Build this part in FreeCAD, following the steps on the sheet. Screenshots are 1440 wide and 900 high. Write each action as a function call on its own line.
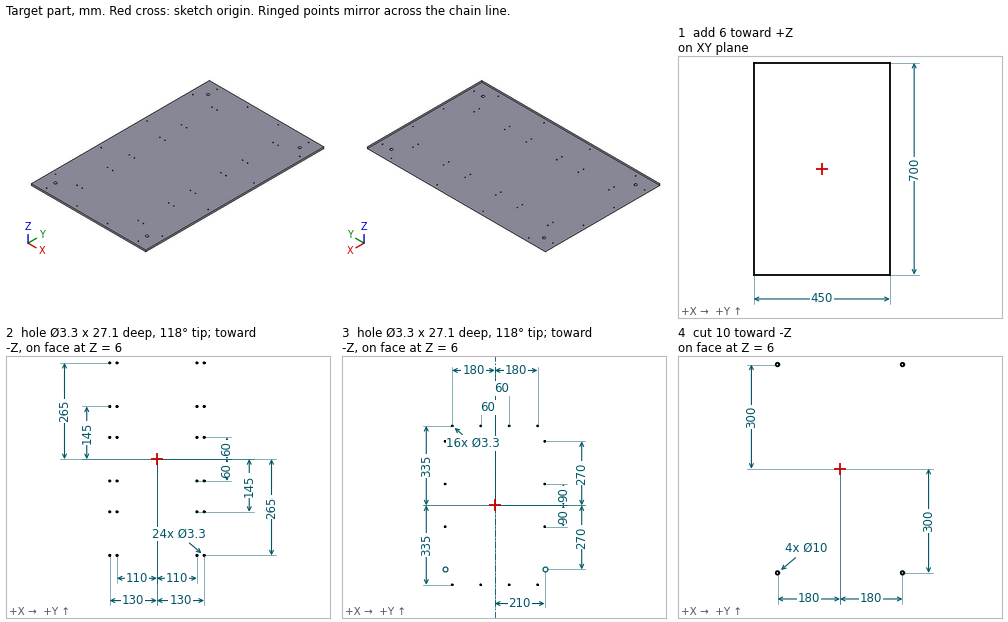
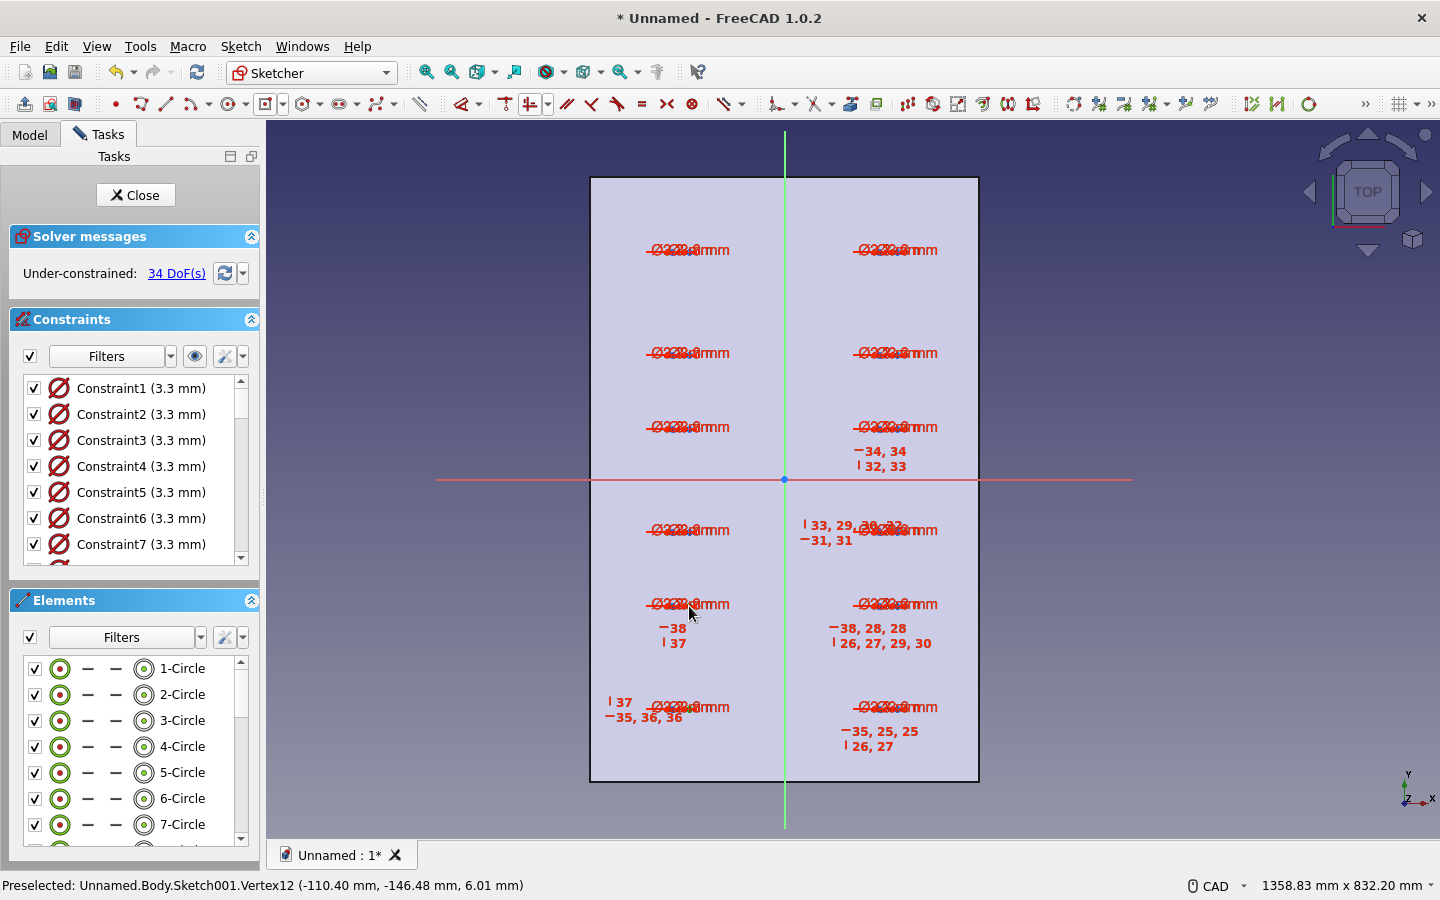
click(548, 104)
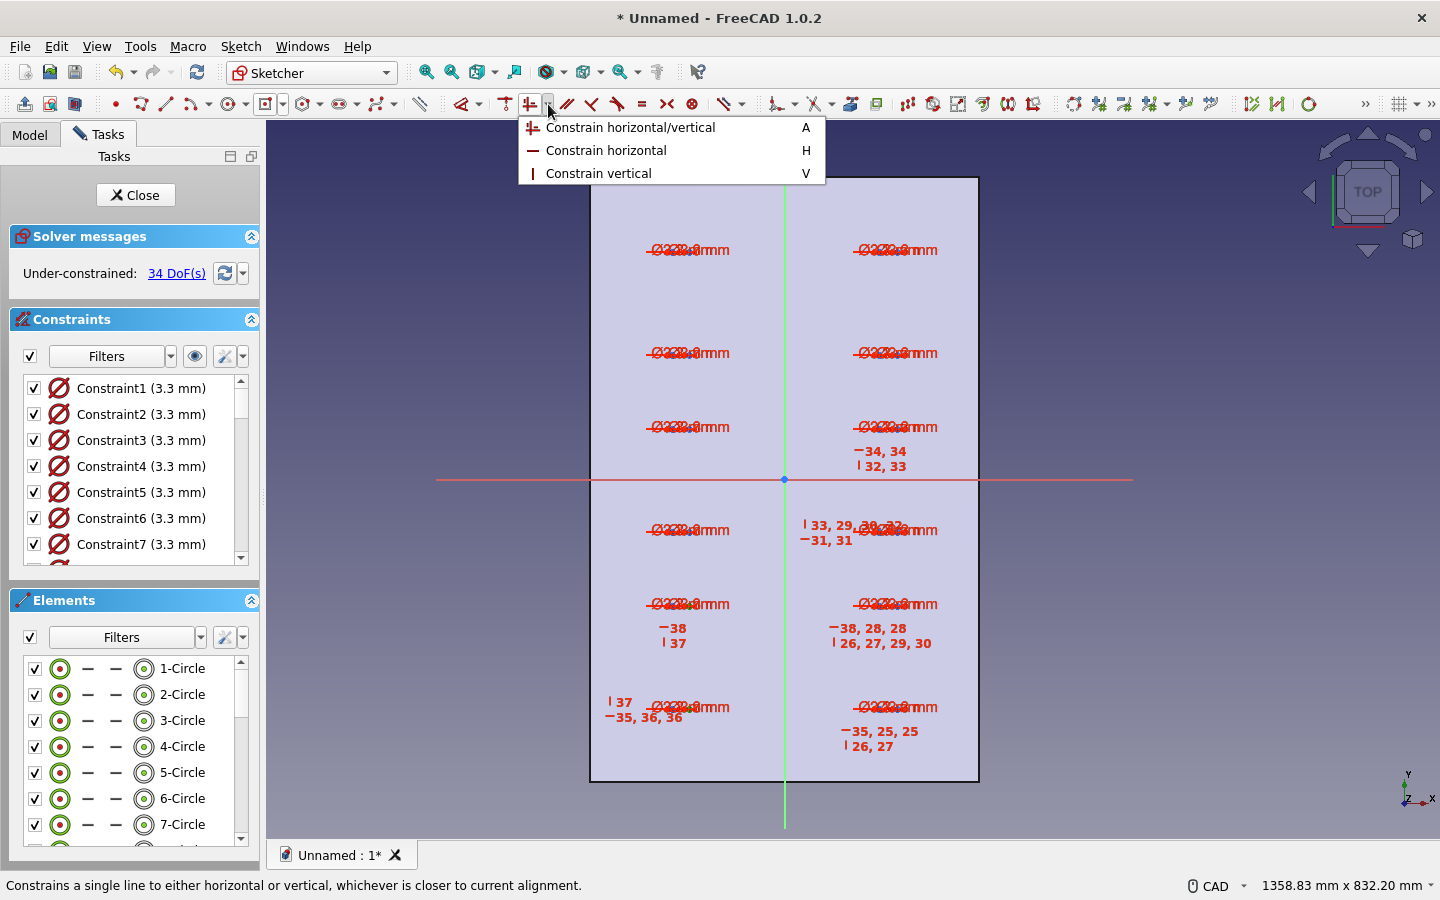
click(672, 174)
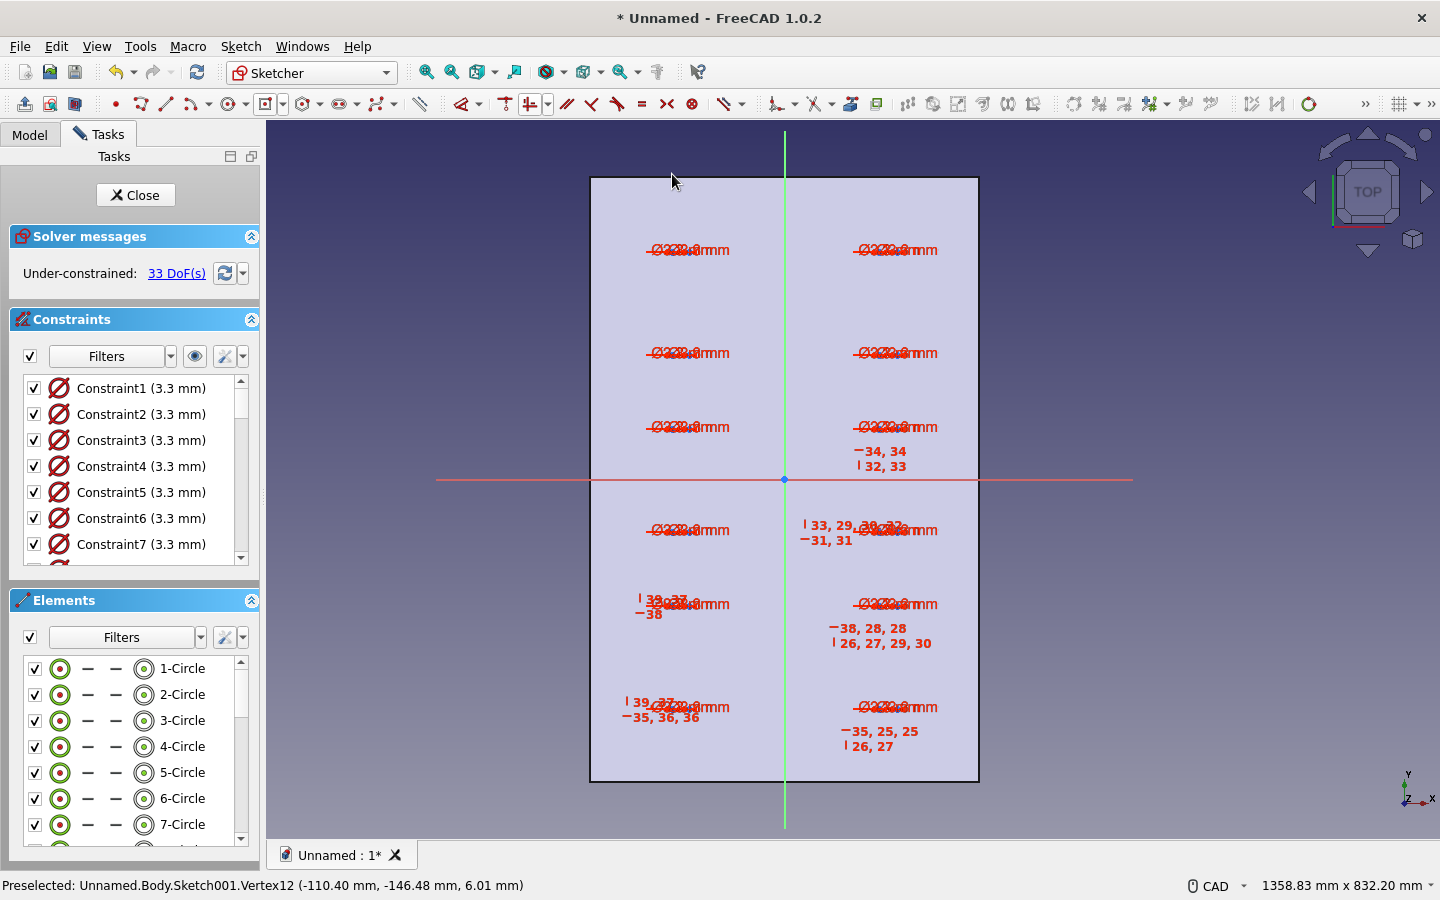
scroll(672, 606, up, 4)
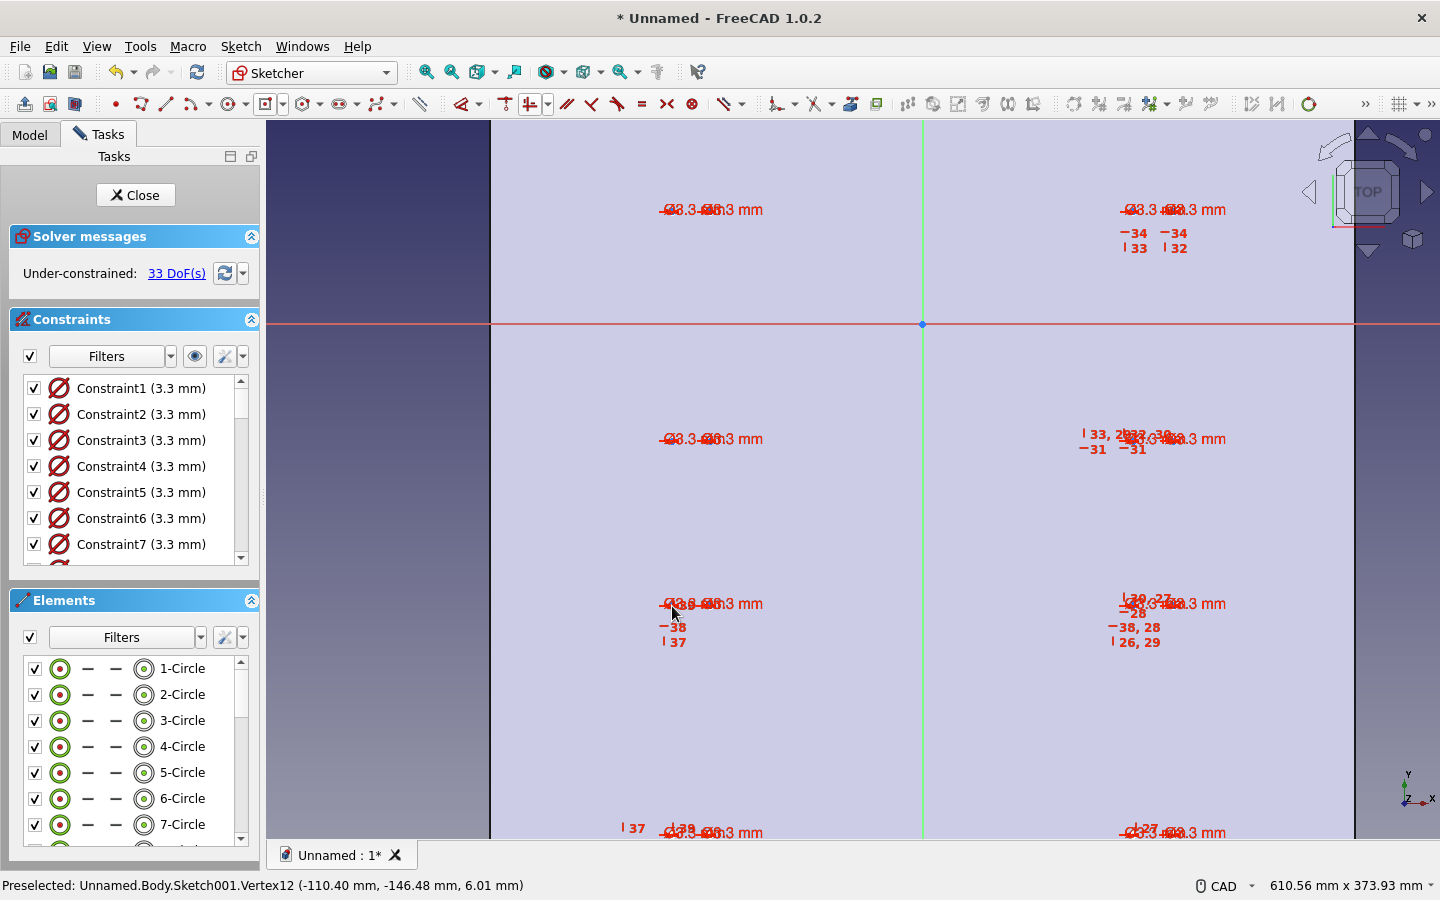
scroll(672, 606, up, 4)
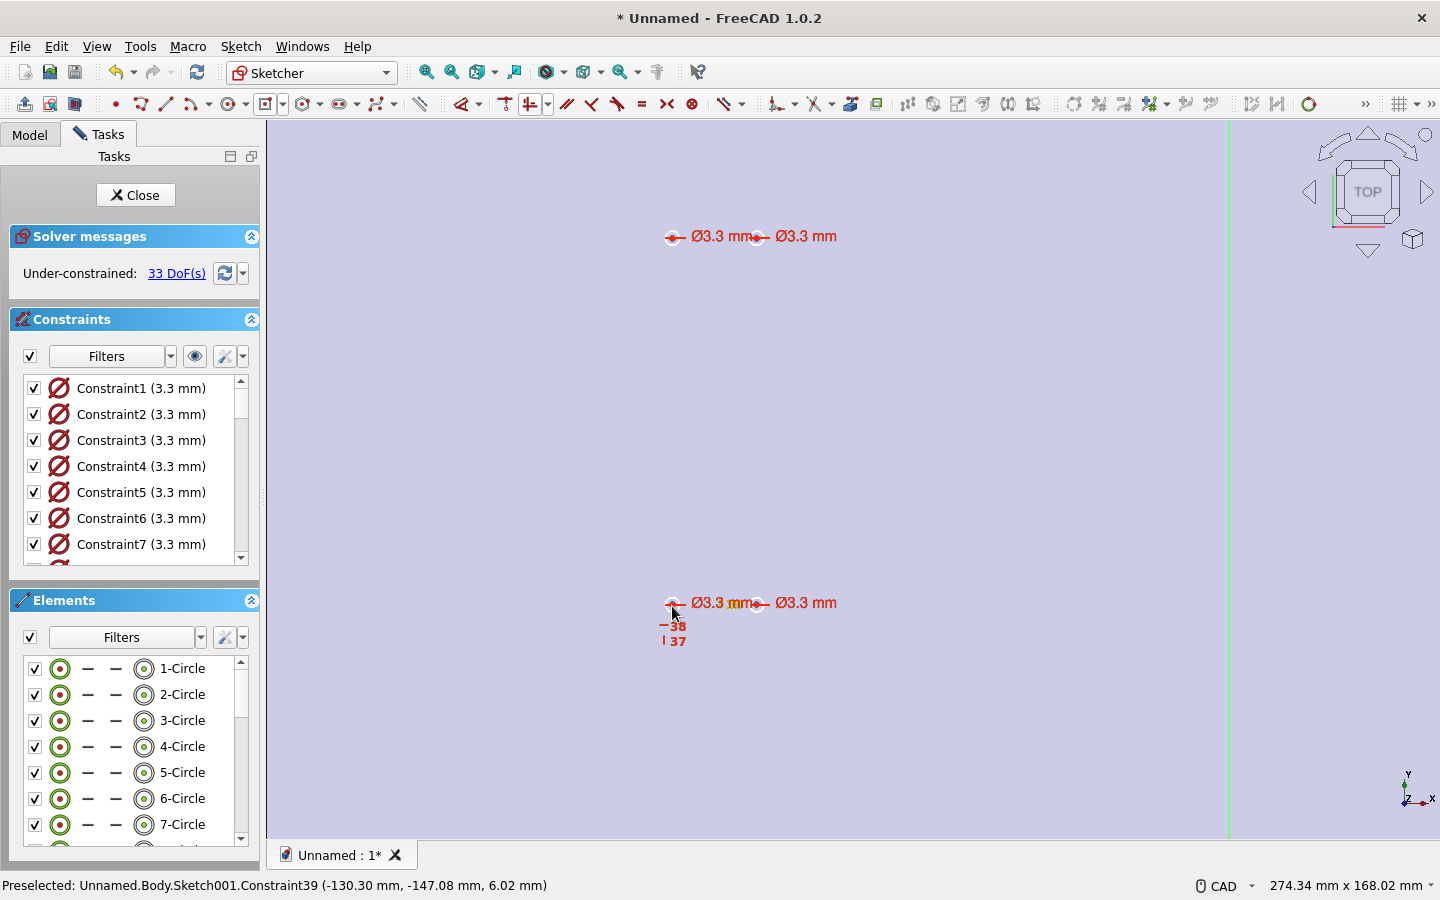
click(673, 605)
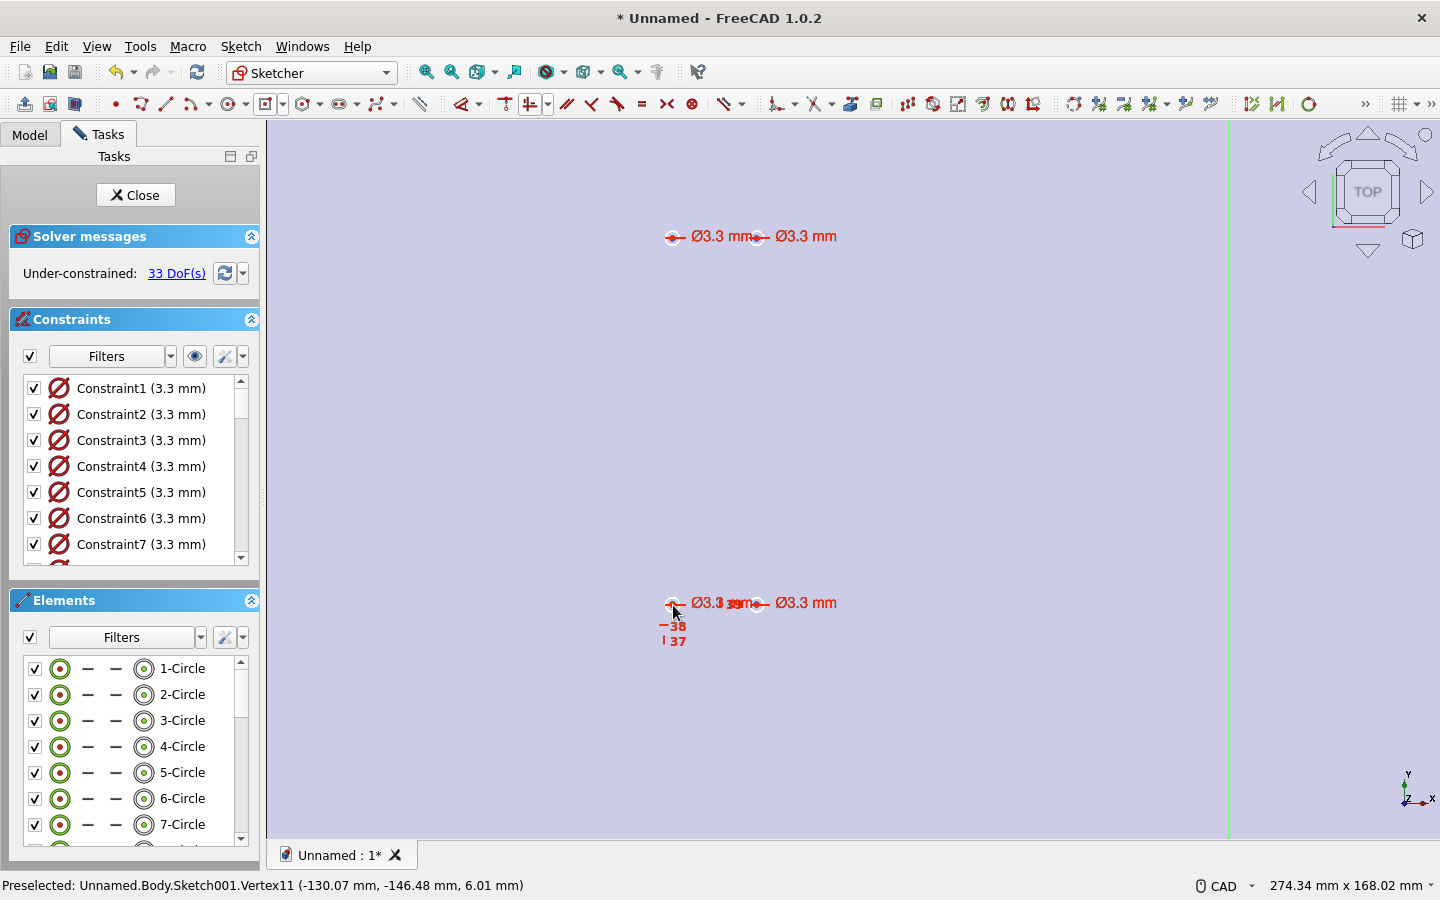
scroll(672, 606, down, 8)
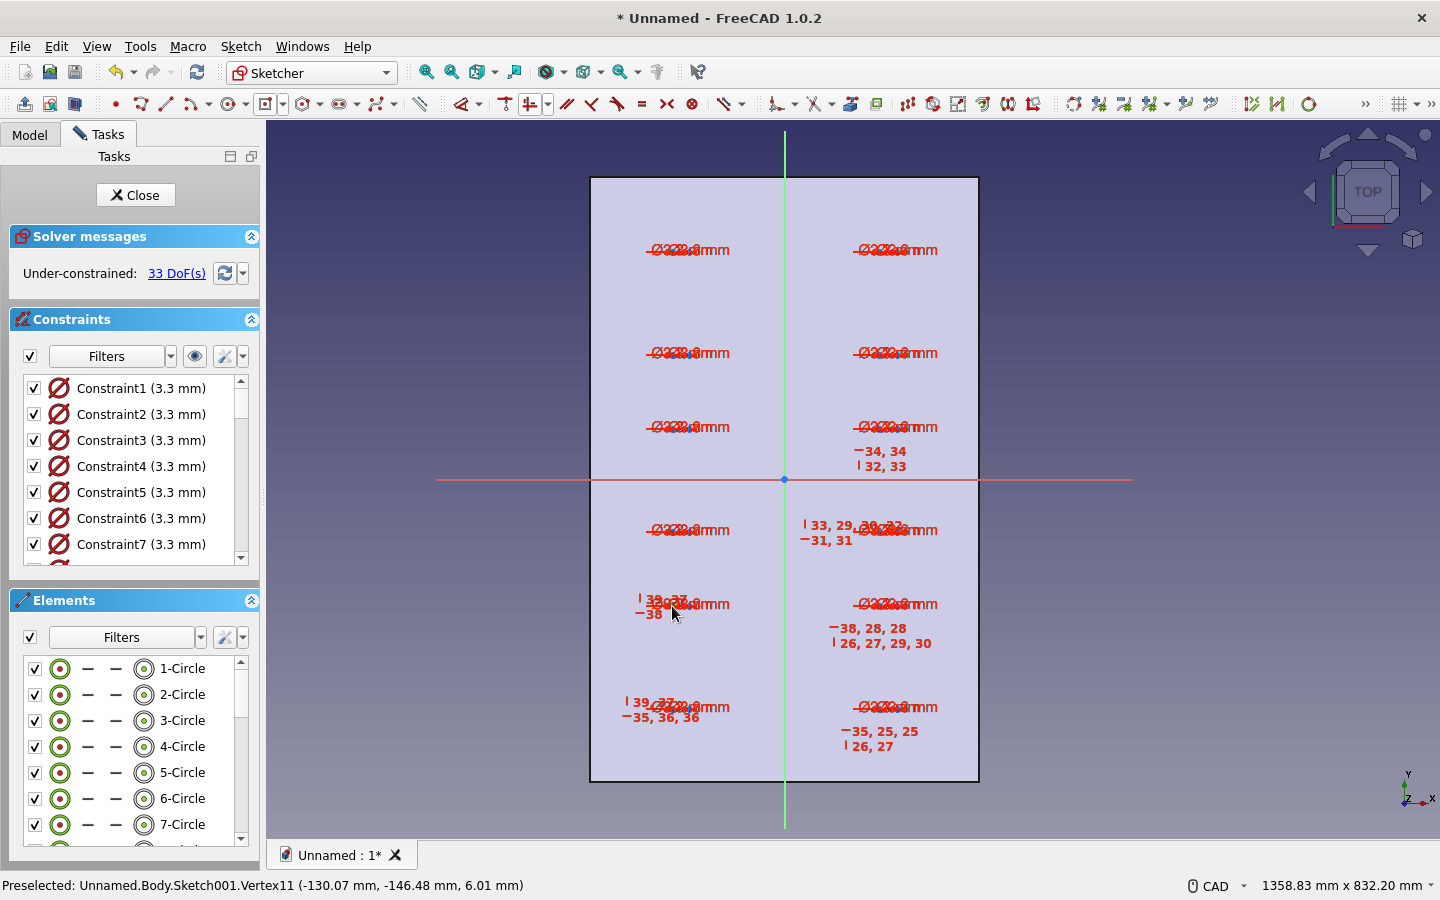
click(689, 606)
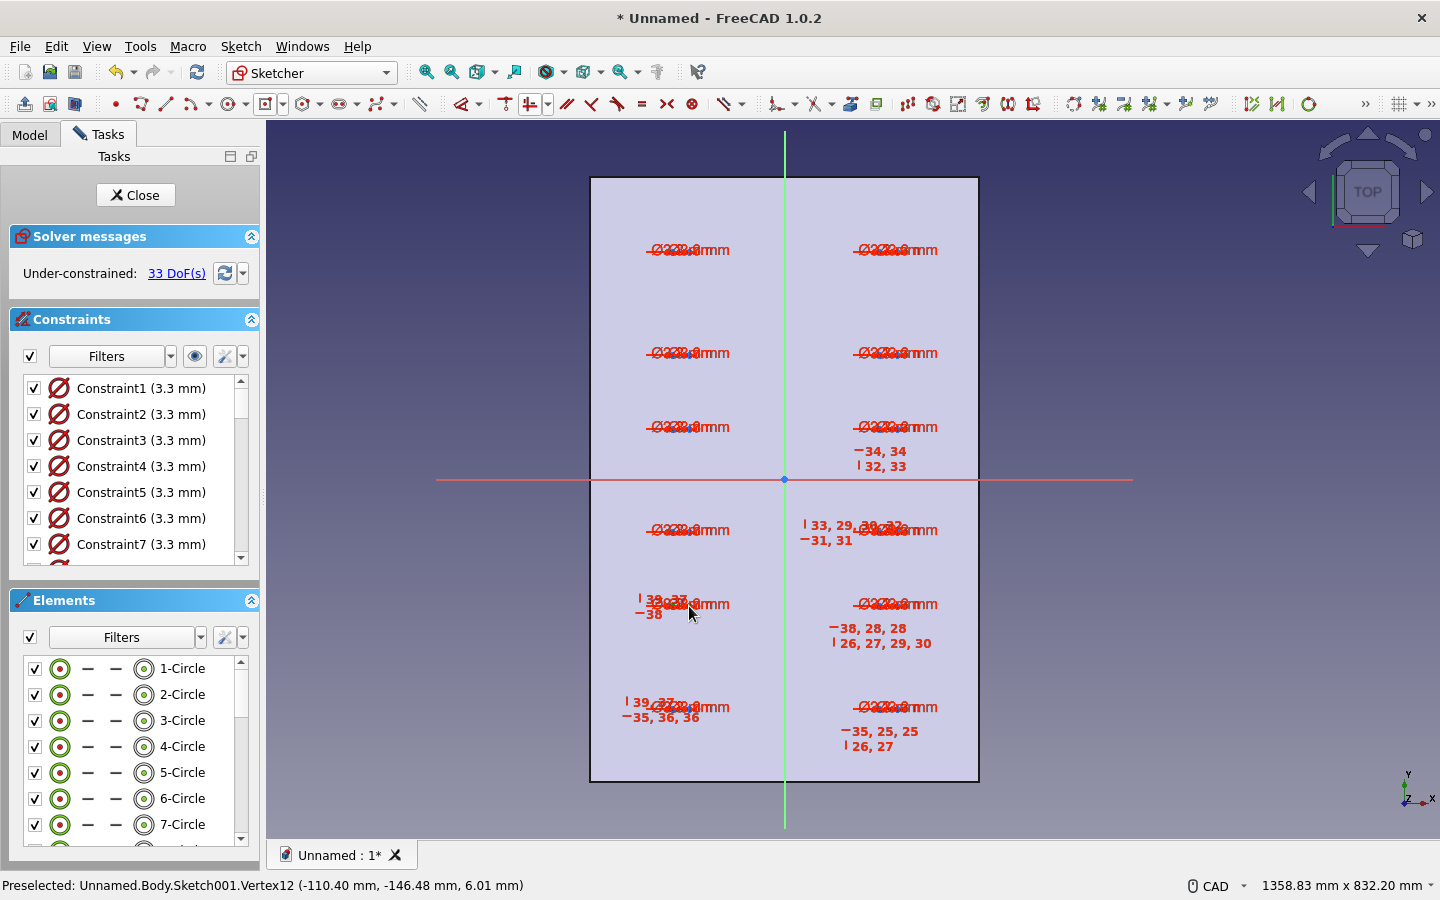
click(548, 104)